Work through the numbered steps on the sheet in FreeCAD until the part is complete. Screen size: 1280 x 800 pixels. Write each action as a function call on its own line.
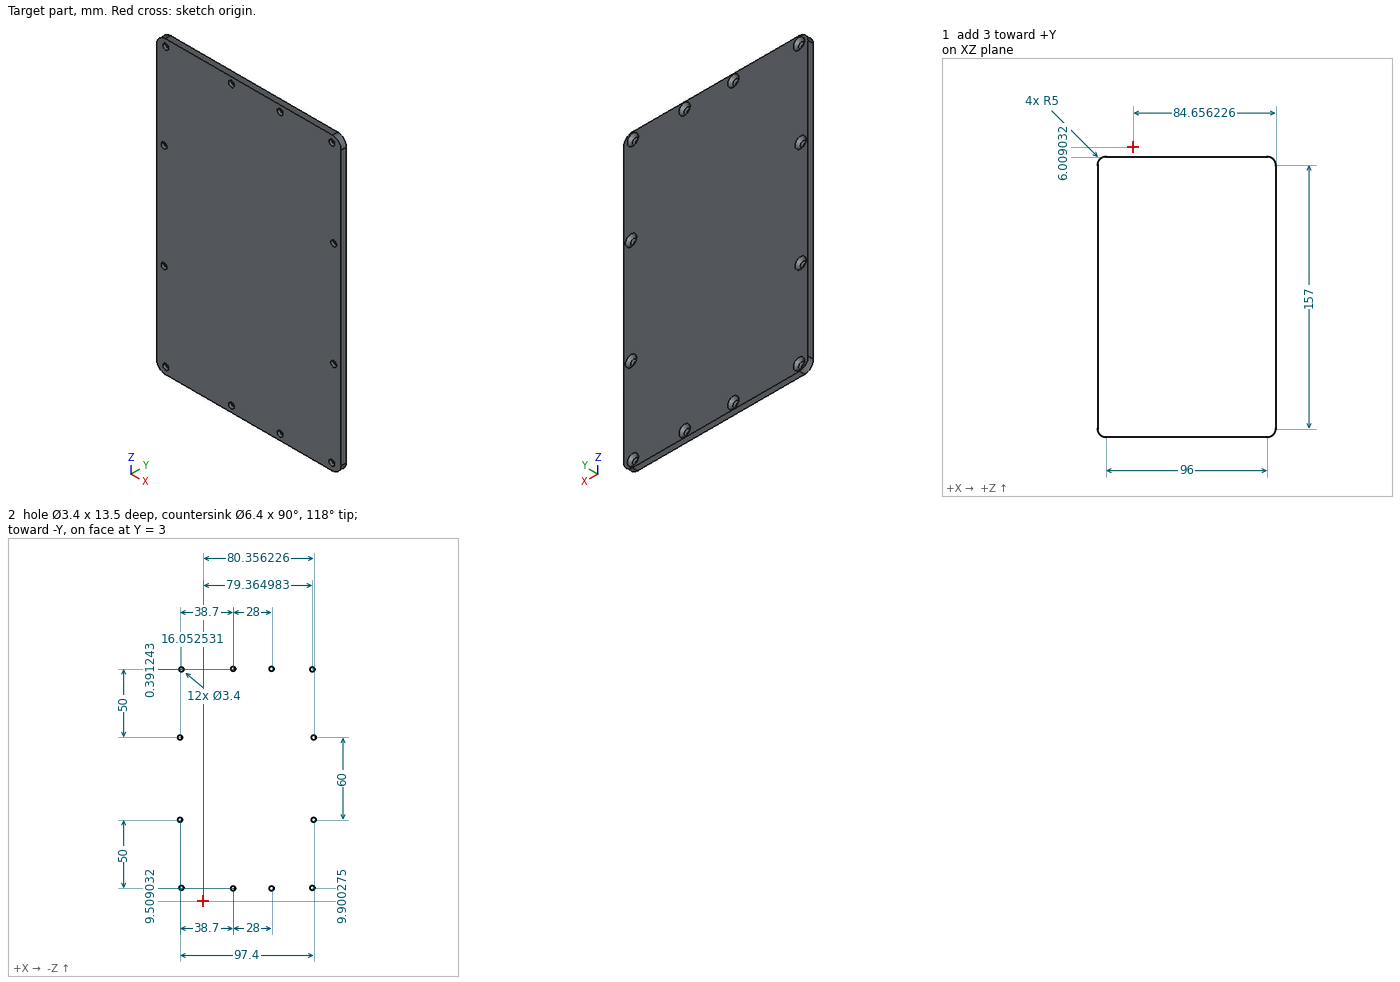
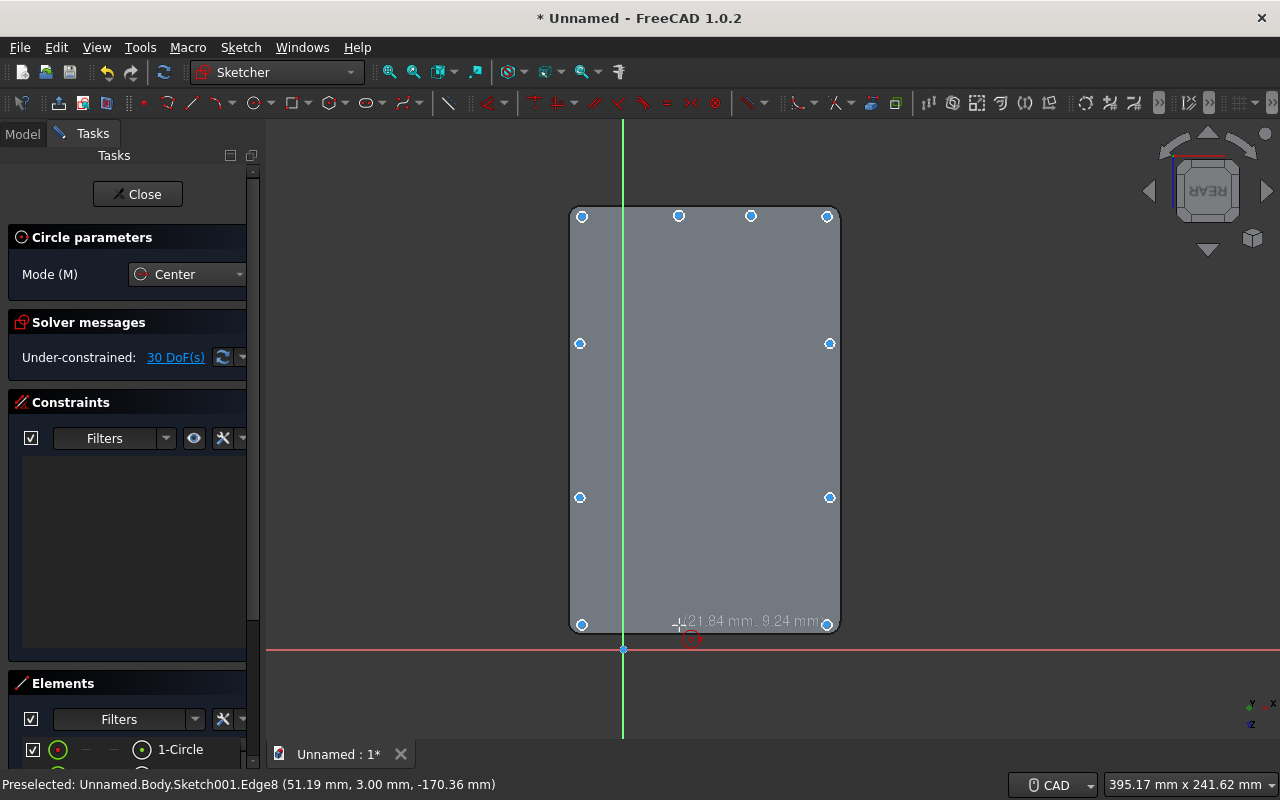
click(679, 625)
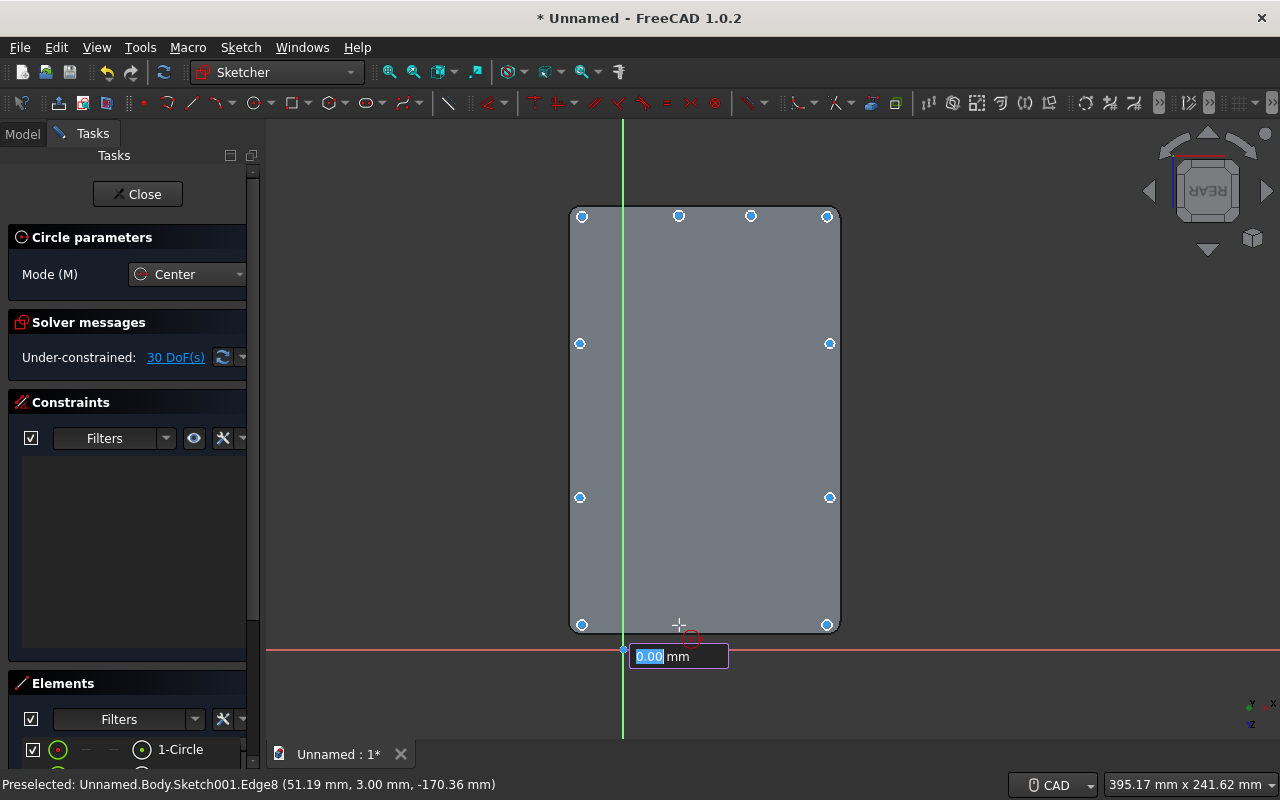
scroll(682, 622, up, 7)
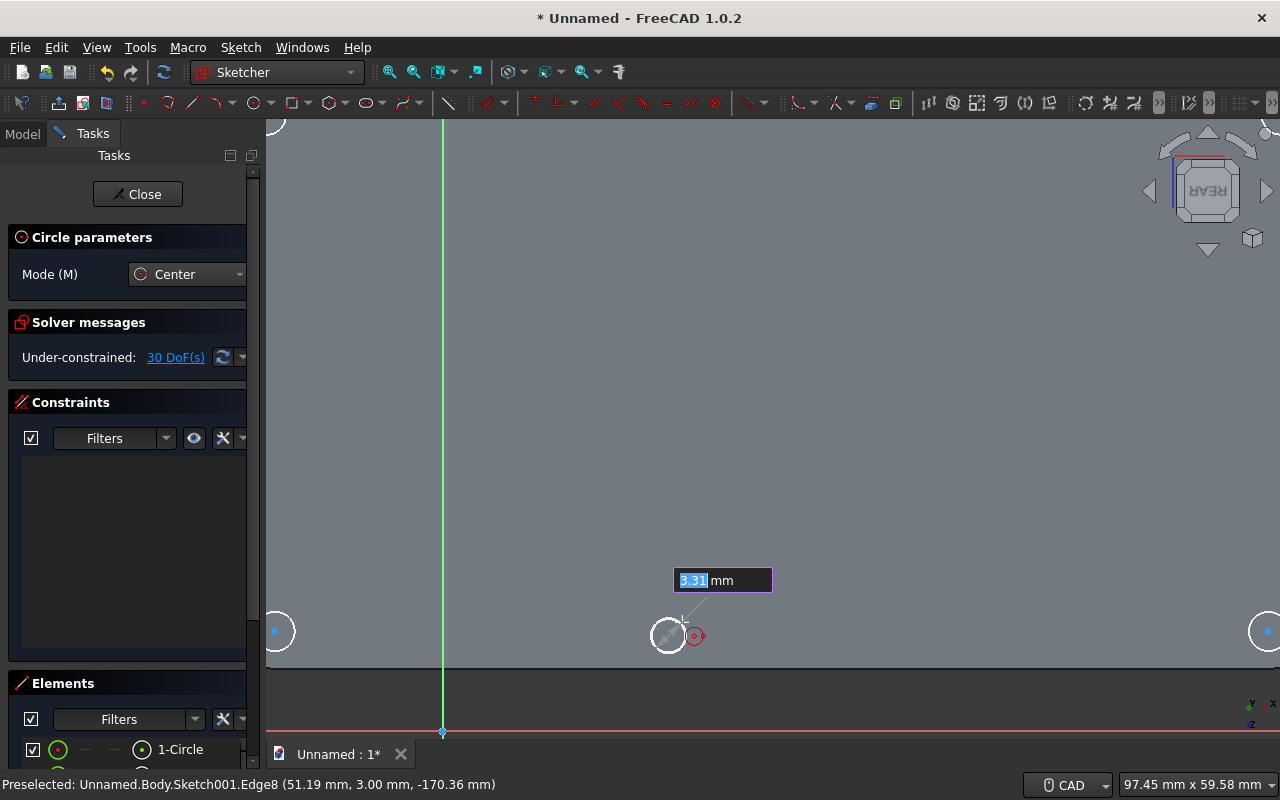
click(681, 620)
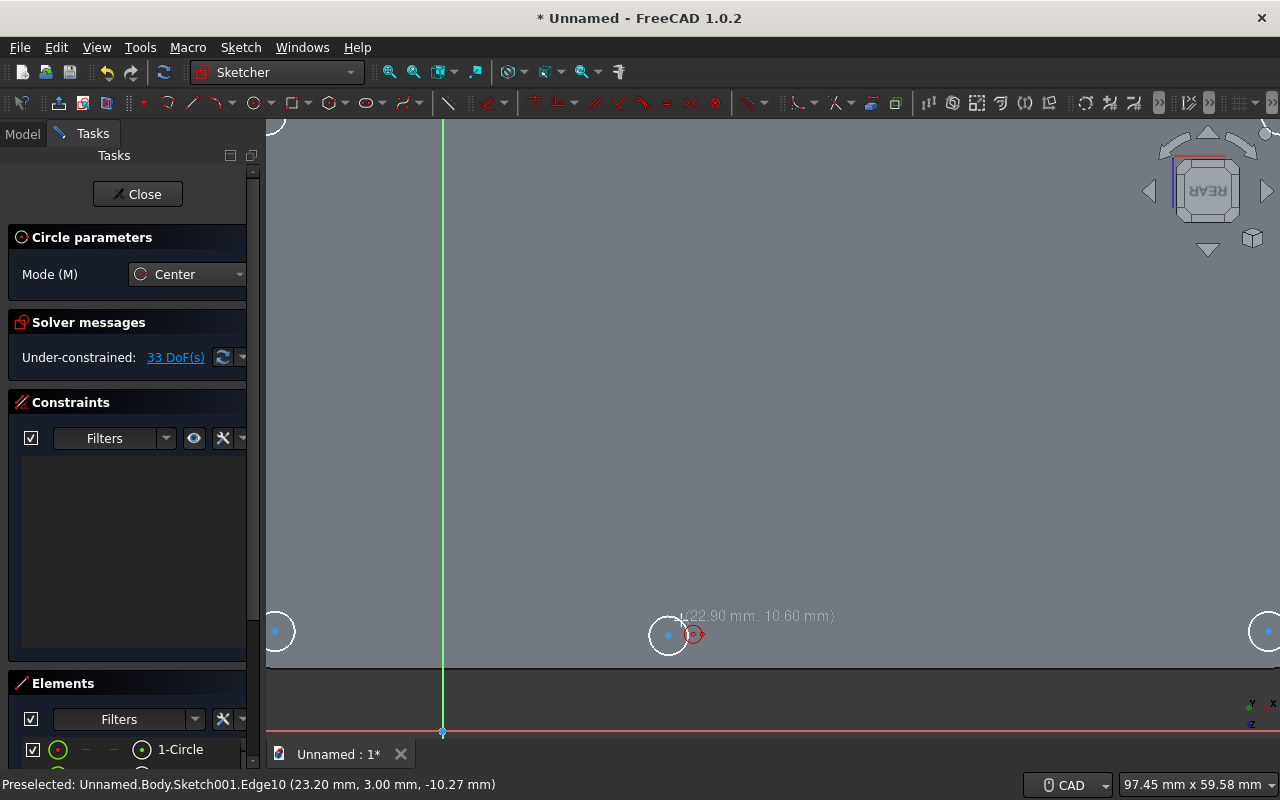
scroll(959, 632, up, 2)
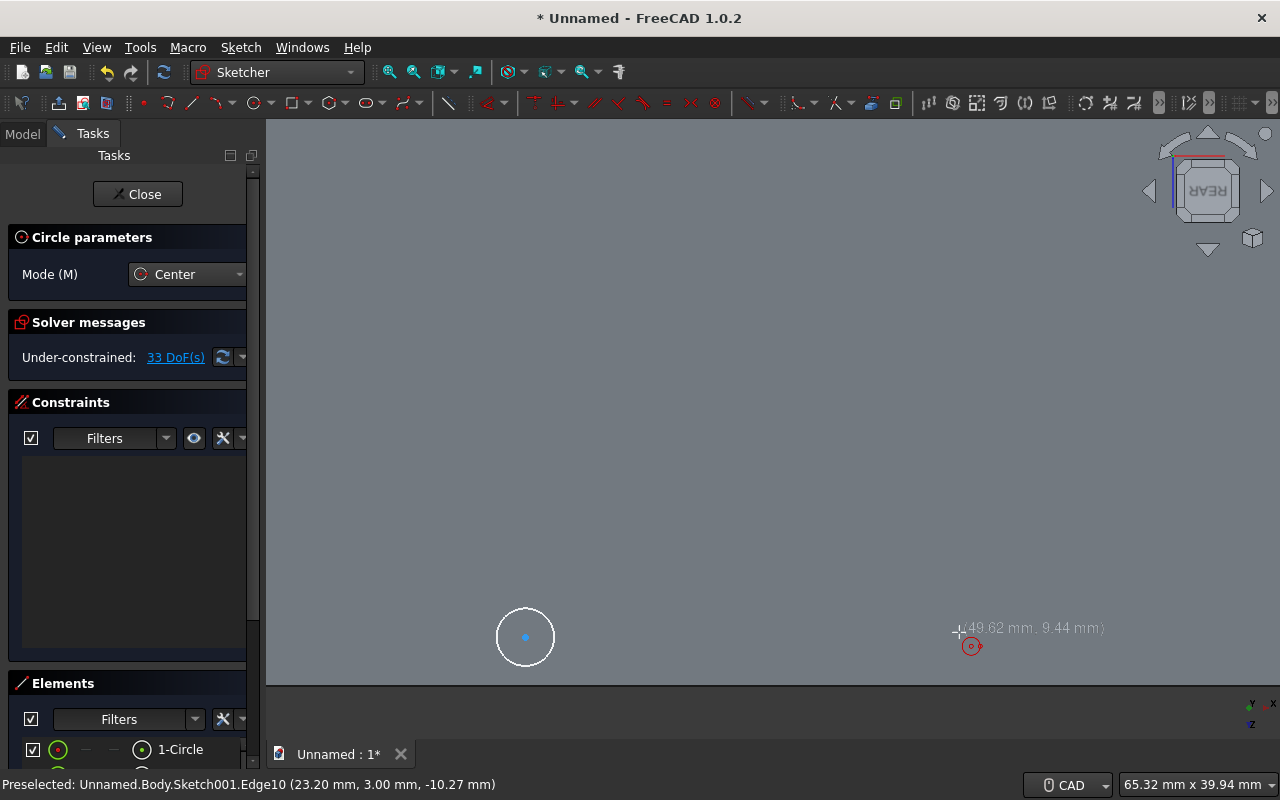
scroll(709, 623, down, 9)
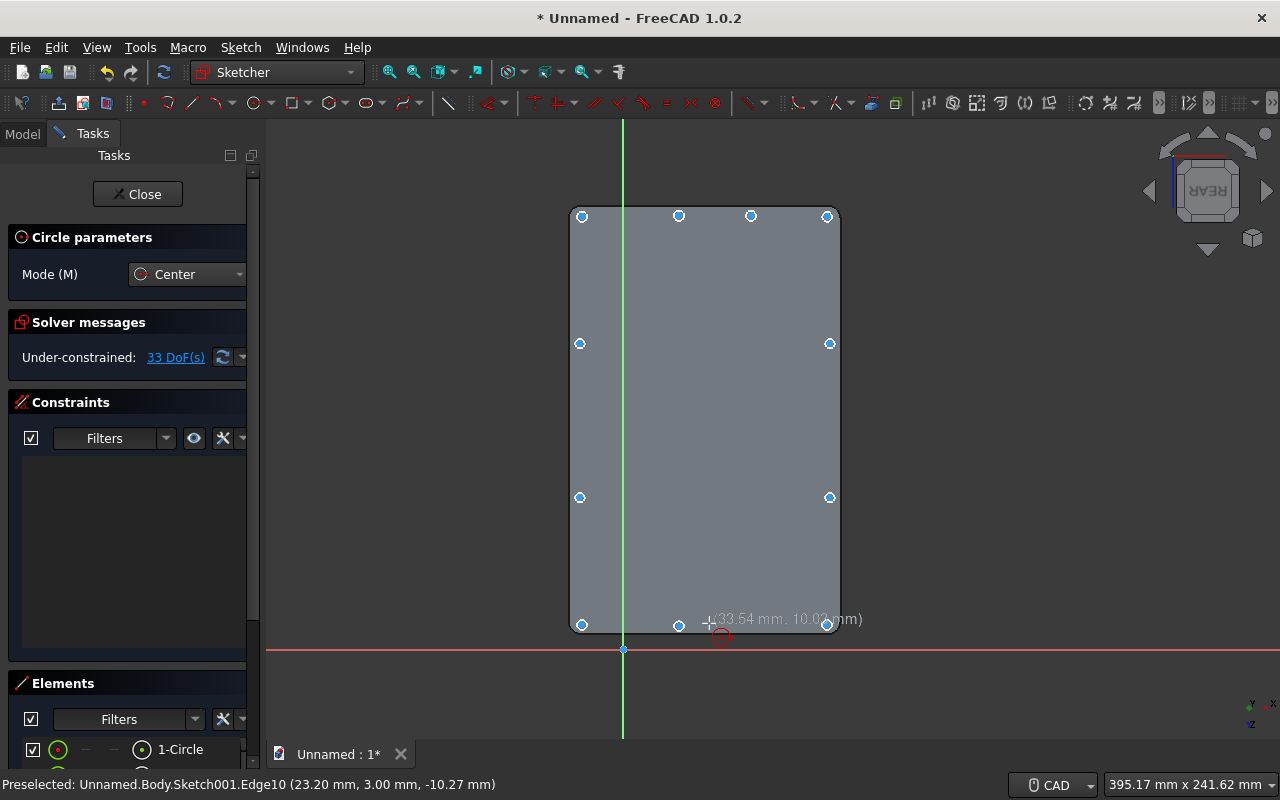
click(751, 625)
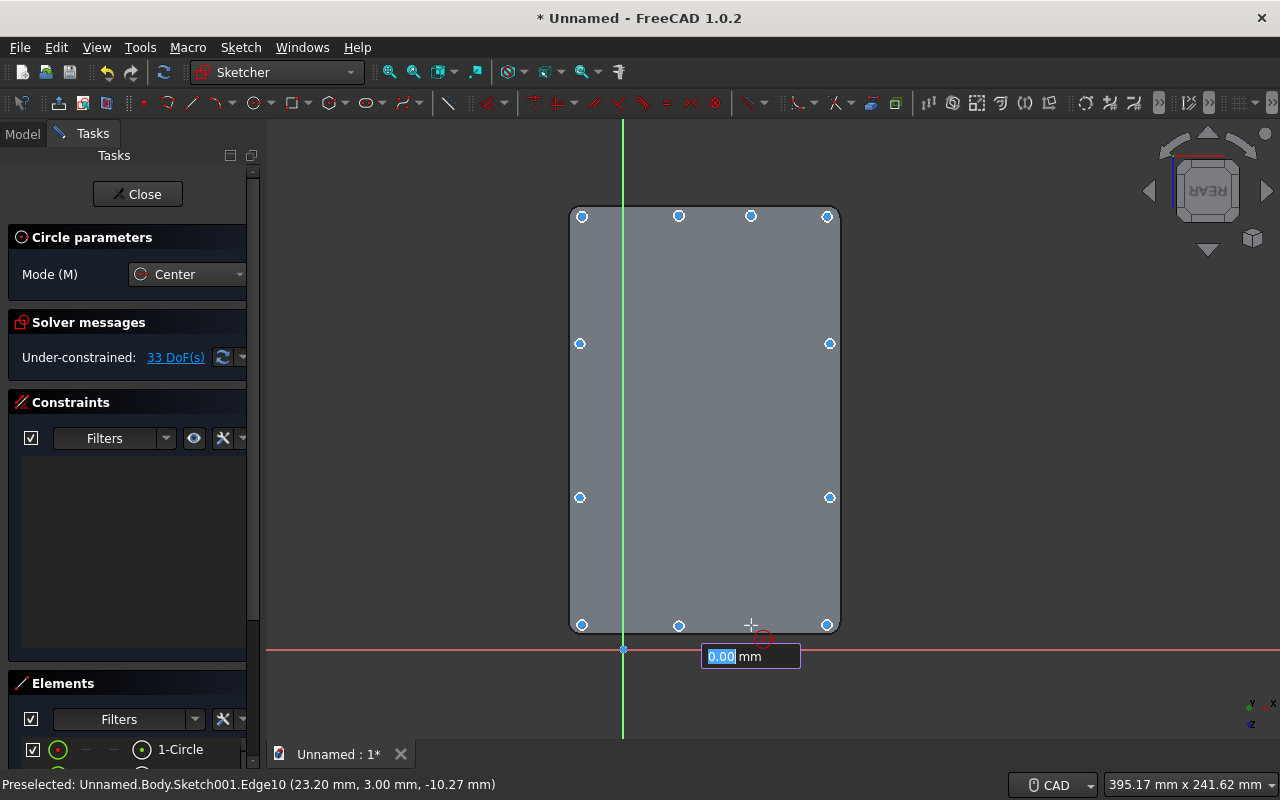
scroll(754, 622, up, 7)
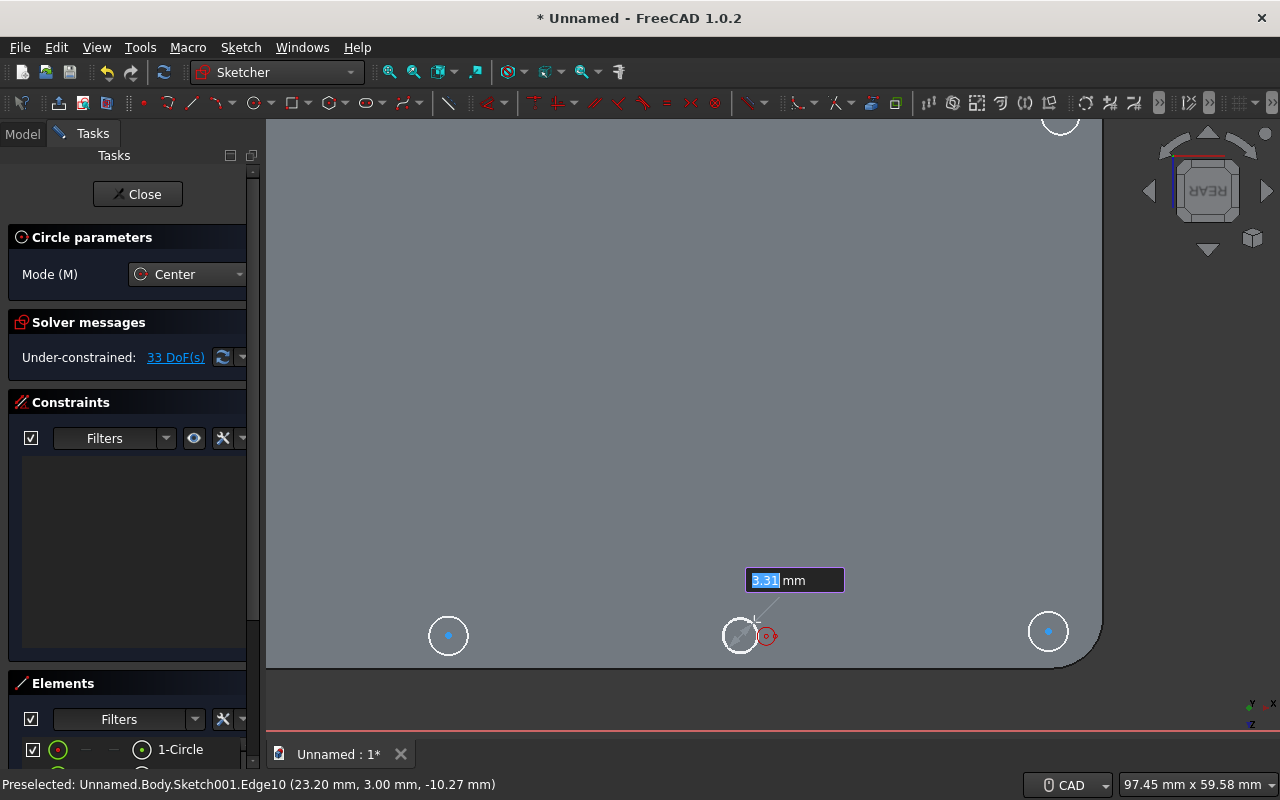
click(752, 620)
key(Escape)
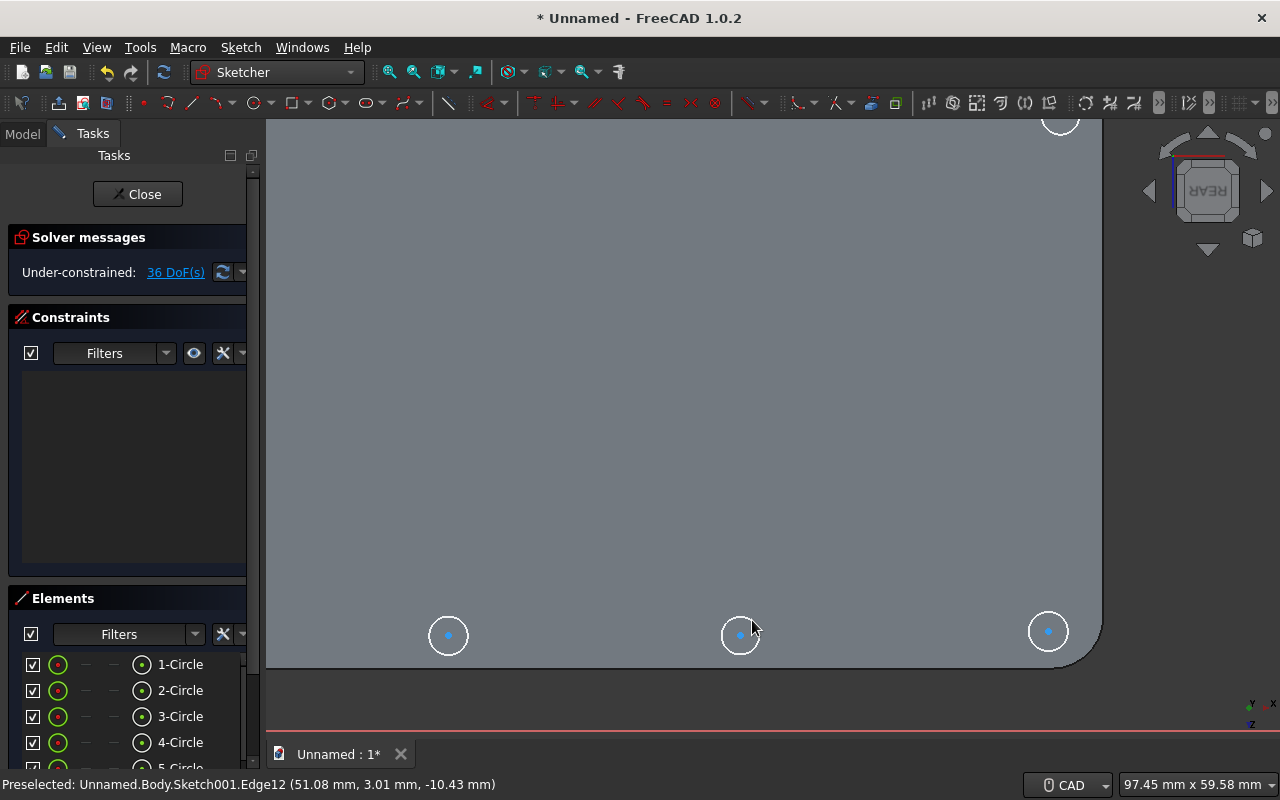
scroll(754, 622, down, 7)